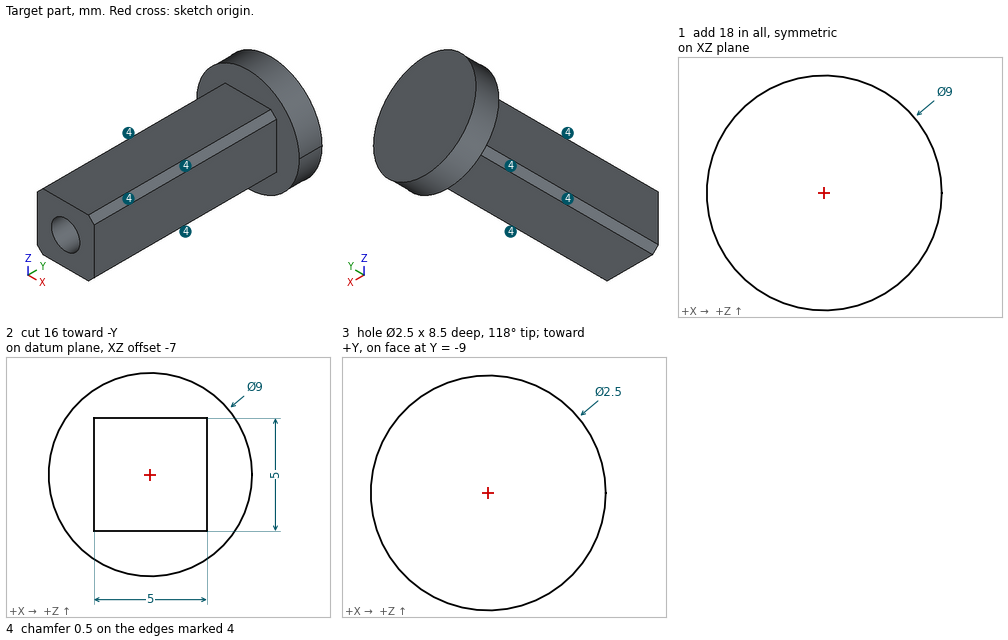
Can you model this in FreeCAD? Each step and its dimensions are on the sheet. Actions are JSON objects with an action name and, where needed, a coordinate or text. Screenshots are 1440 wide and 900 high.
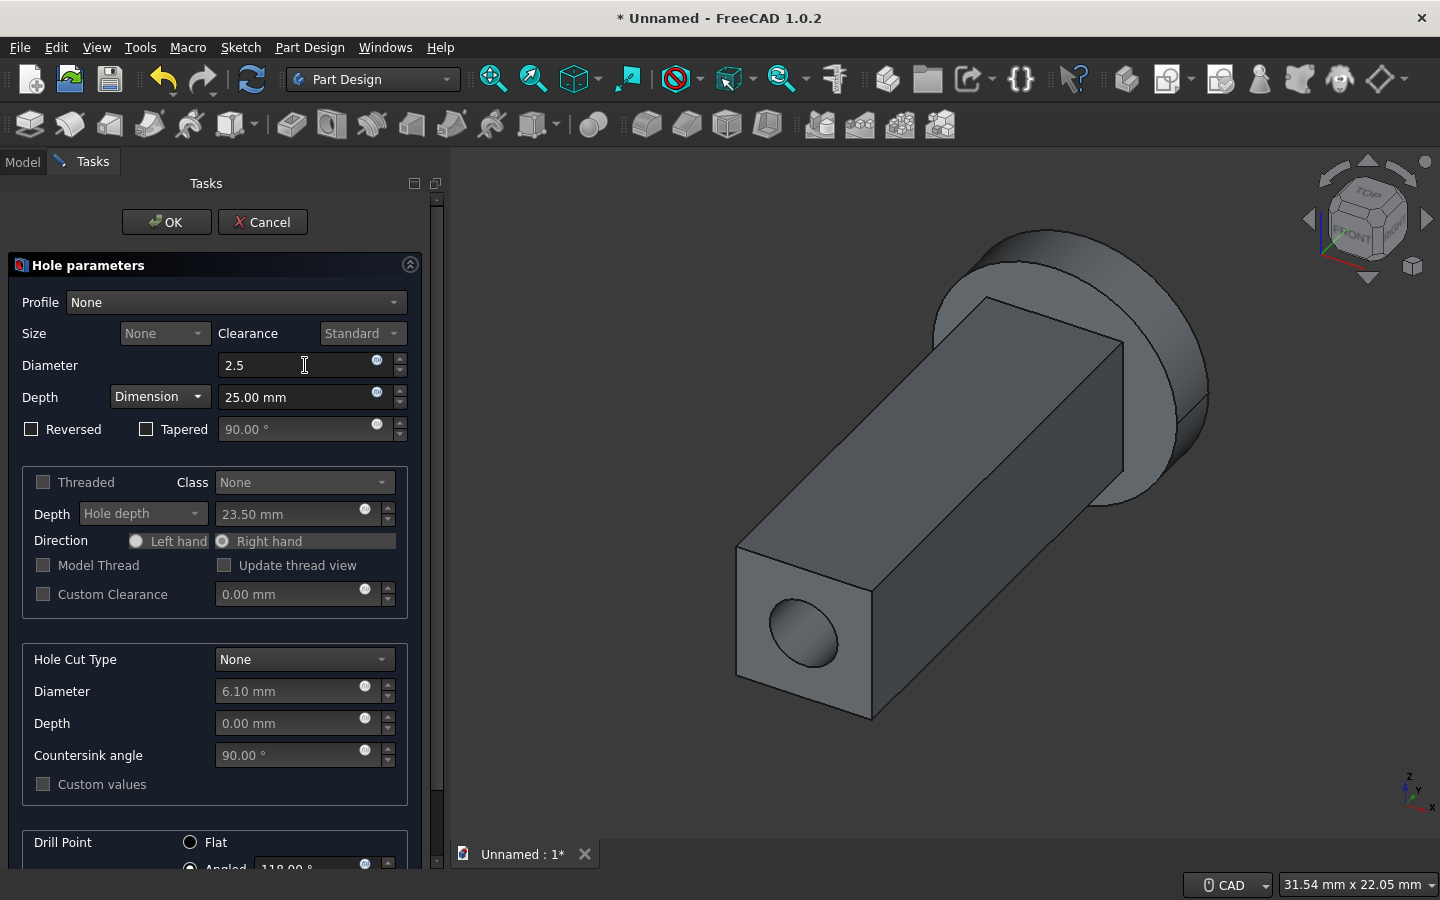
{"action": "triple_click", "coordinate": [305, 397]}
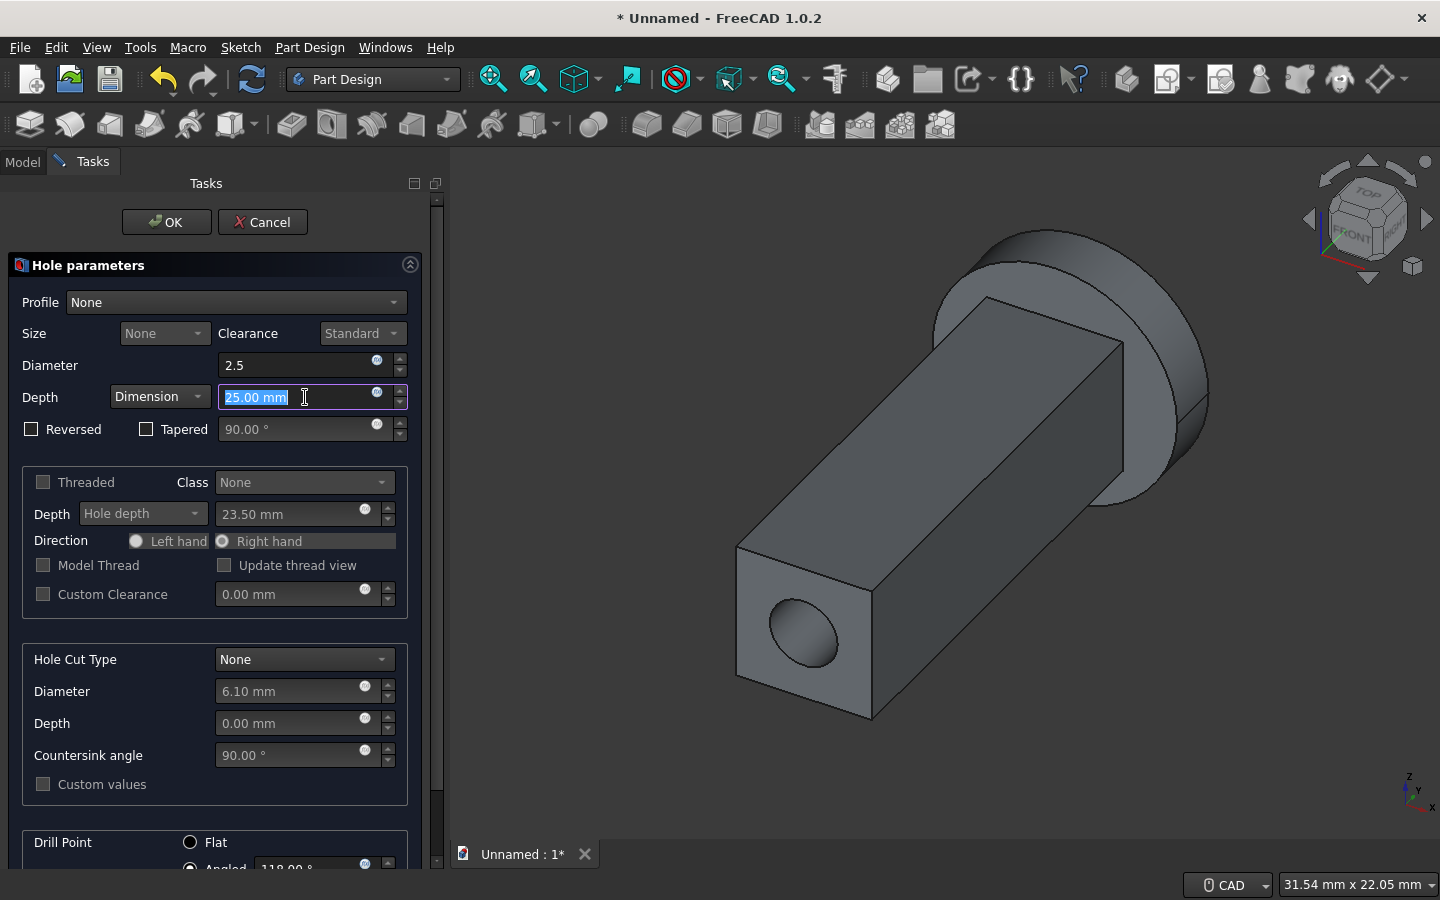
{"action": "type", "text": "8.5"}
{"action": "key", "text": "Tab"}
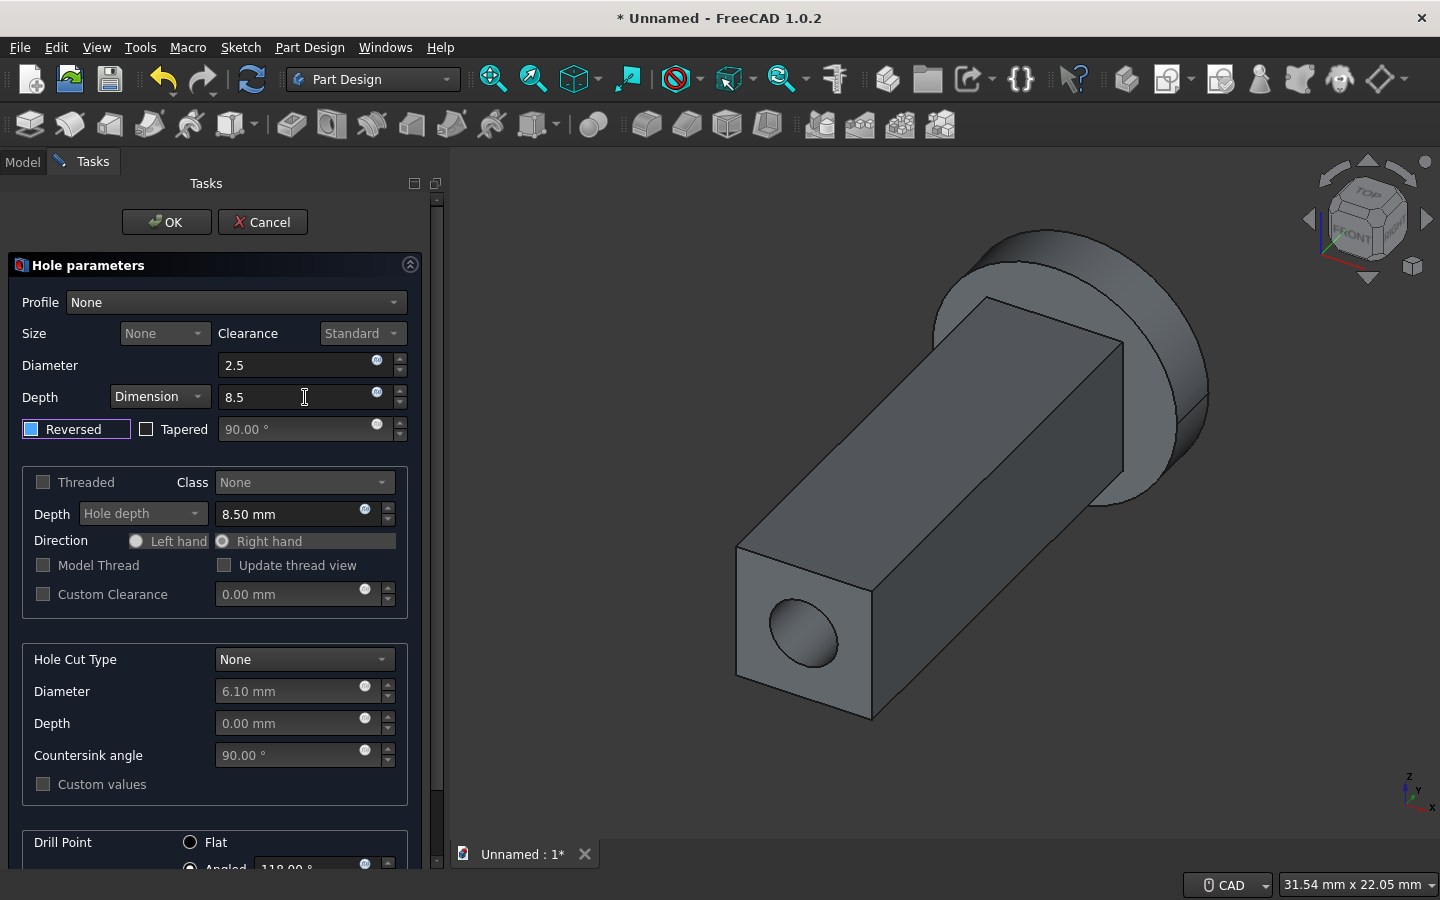
{"action": "left_click", "coordinate": [167, 222]}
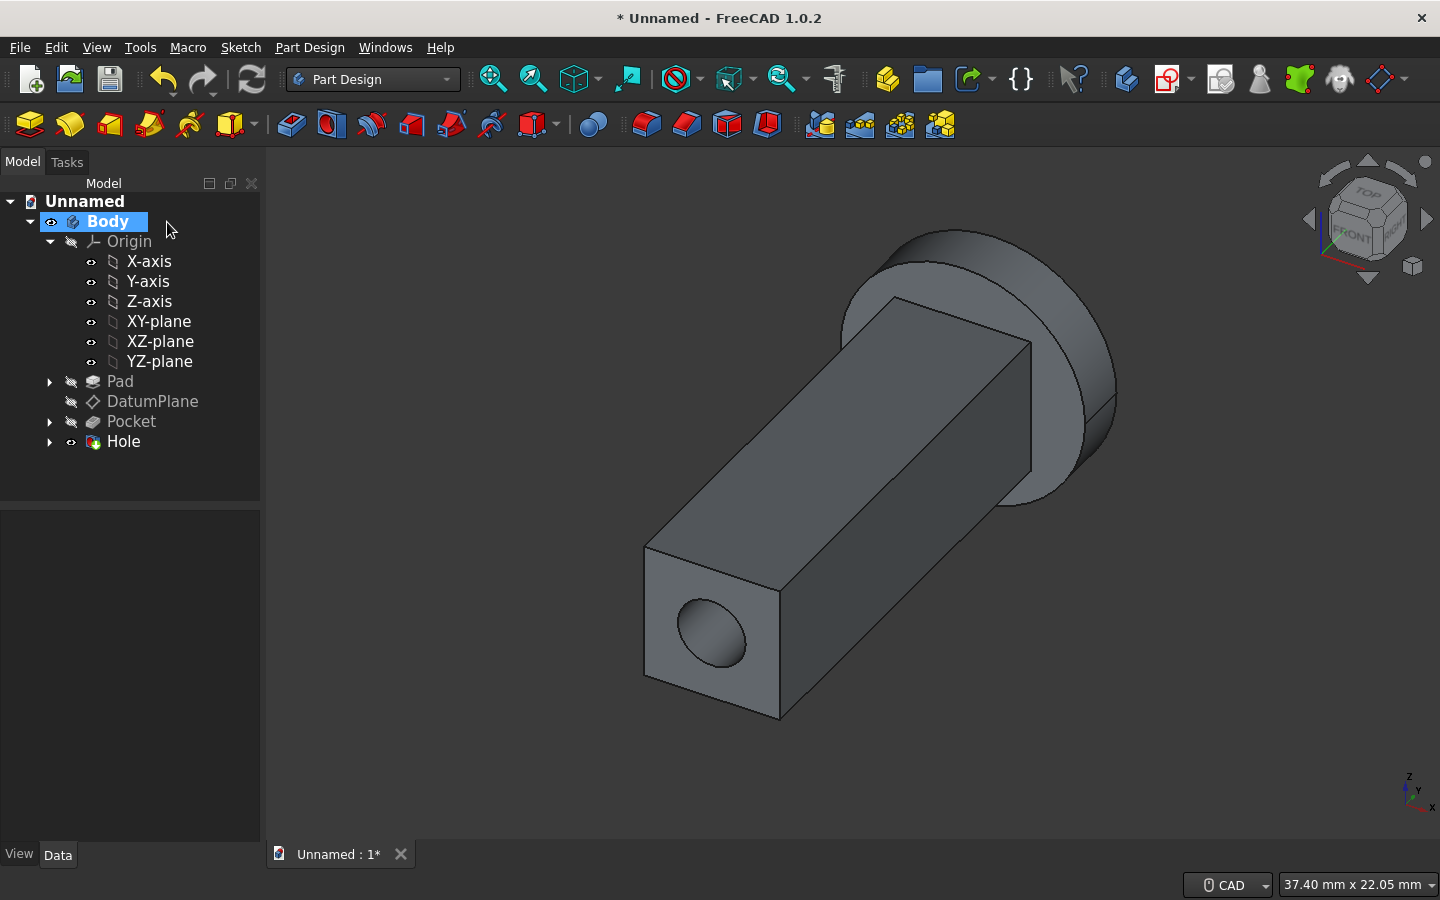
{"action": "left_click", "coordinate": [905, 466]}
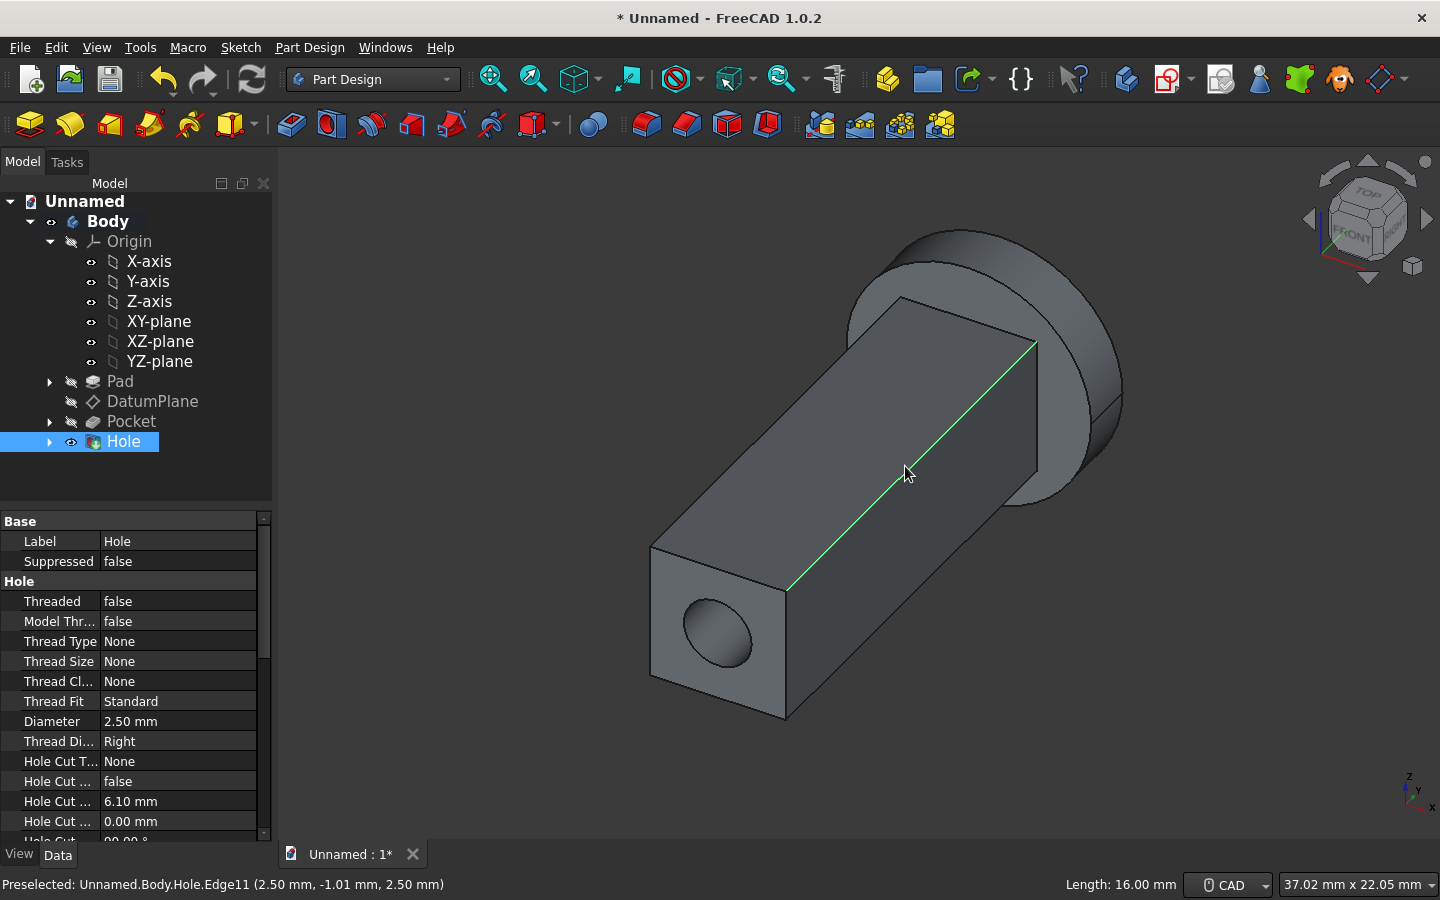
{"action": "key", "text": "0"}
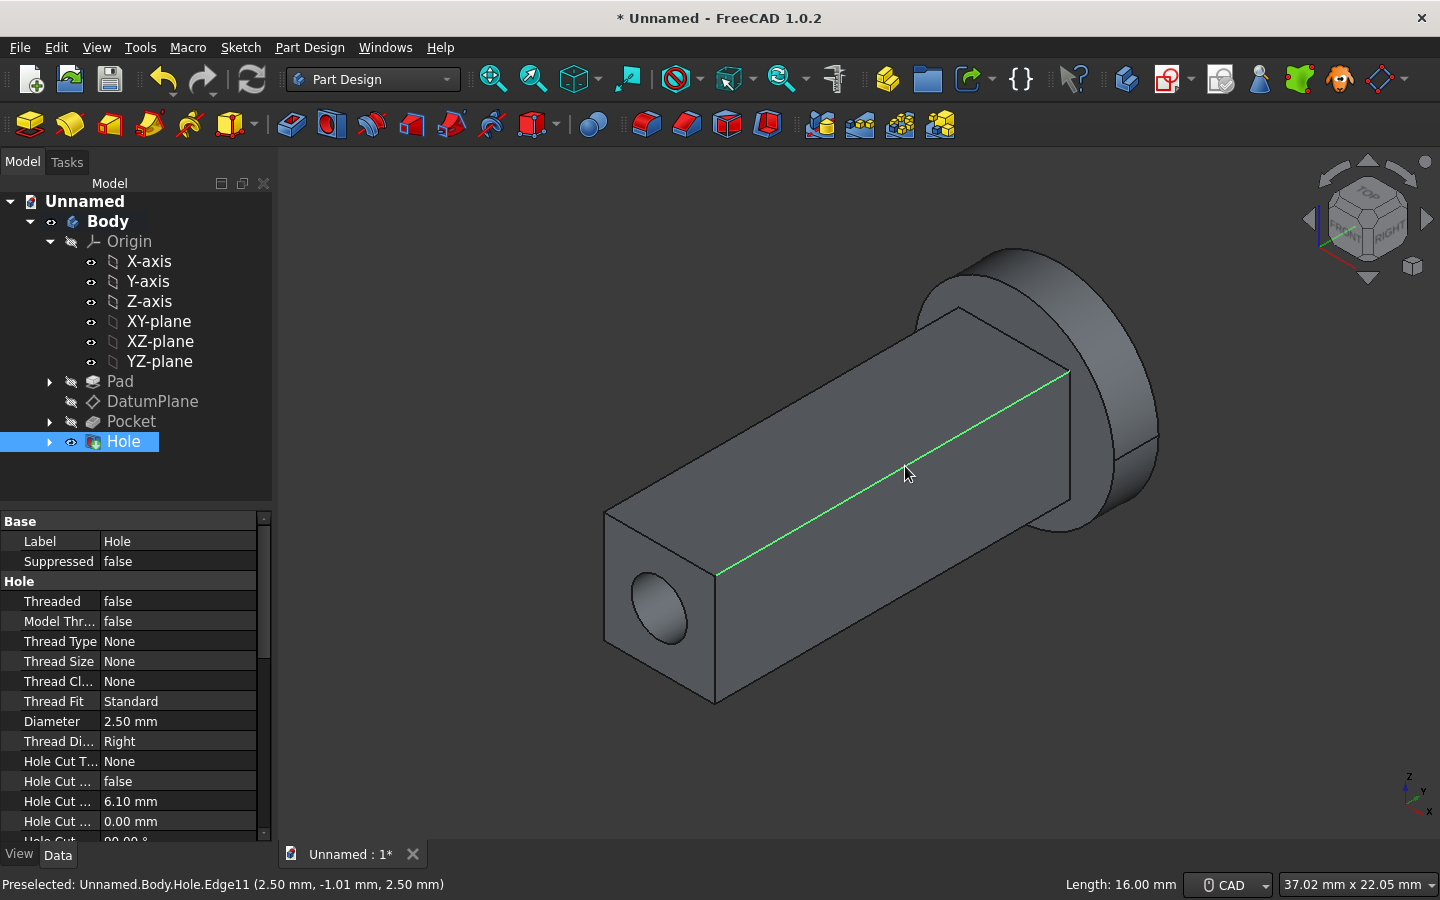
{"action": "key", "text": "2"}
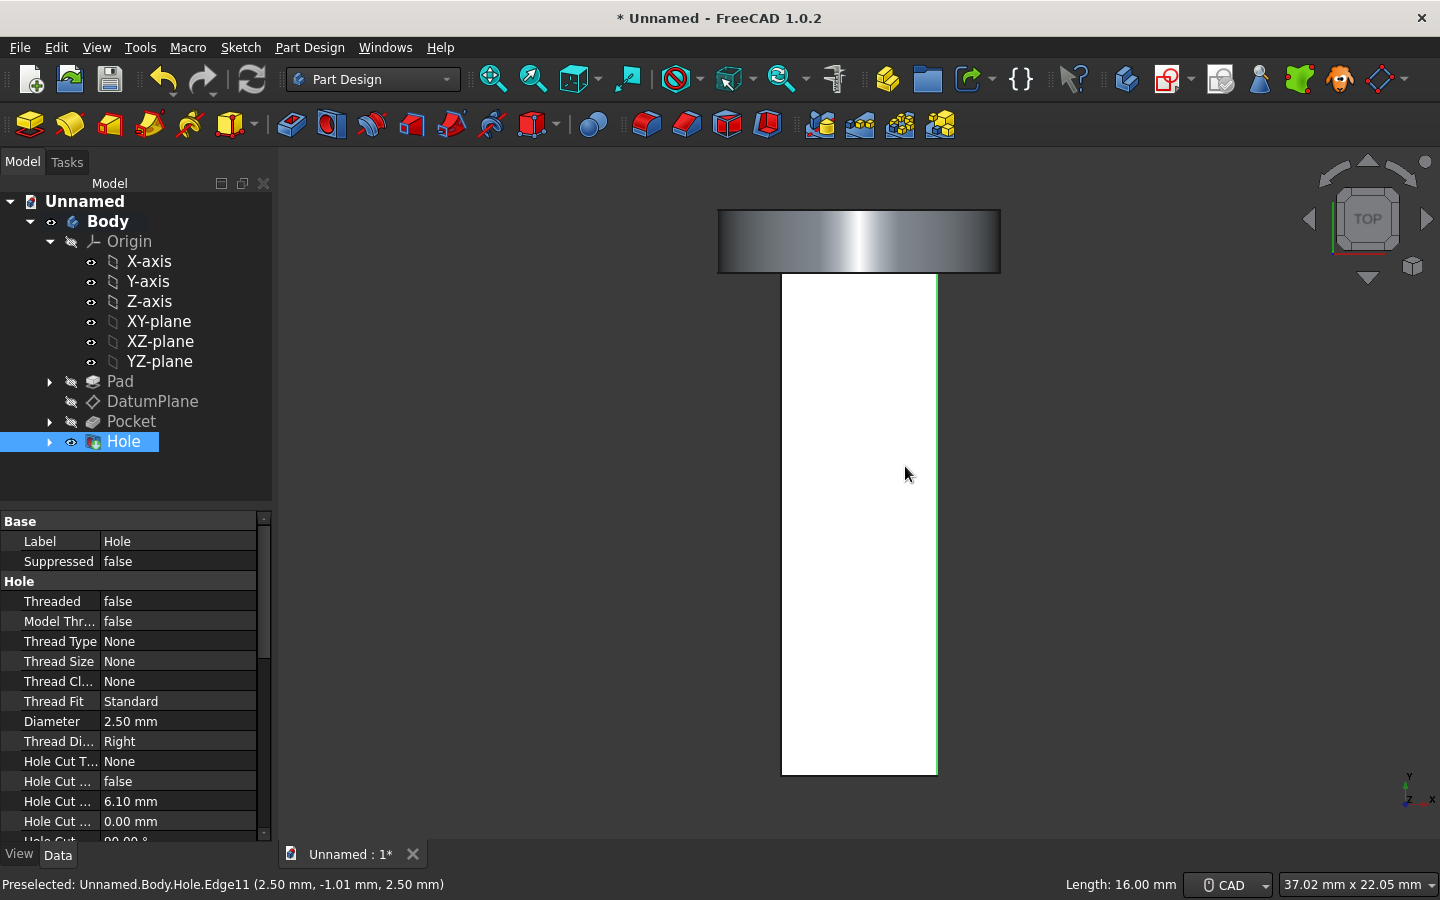
{"action": "left_click", "coordinate": [781, 523], "text": "ctrl"}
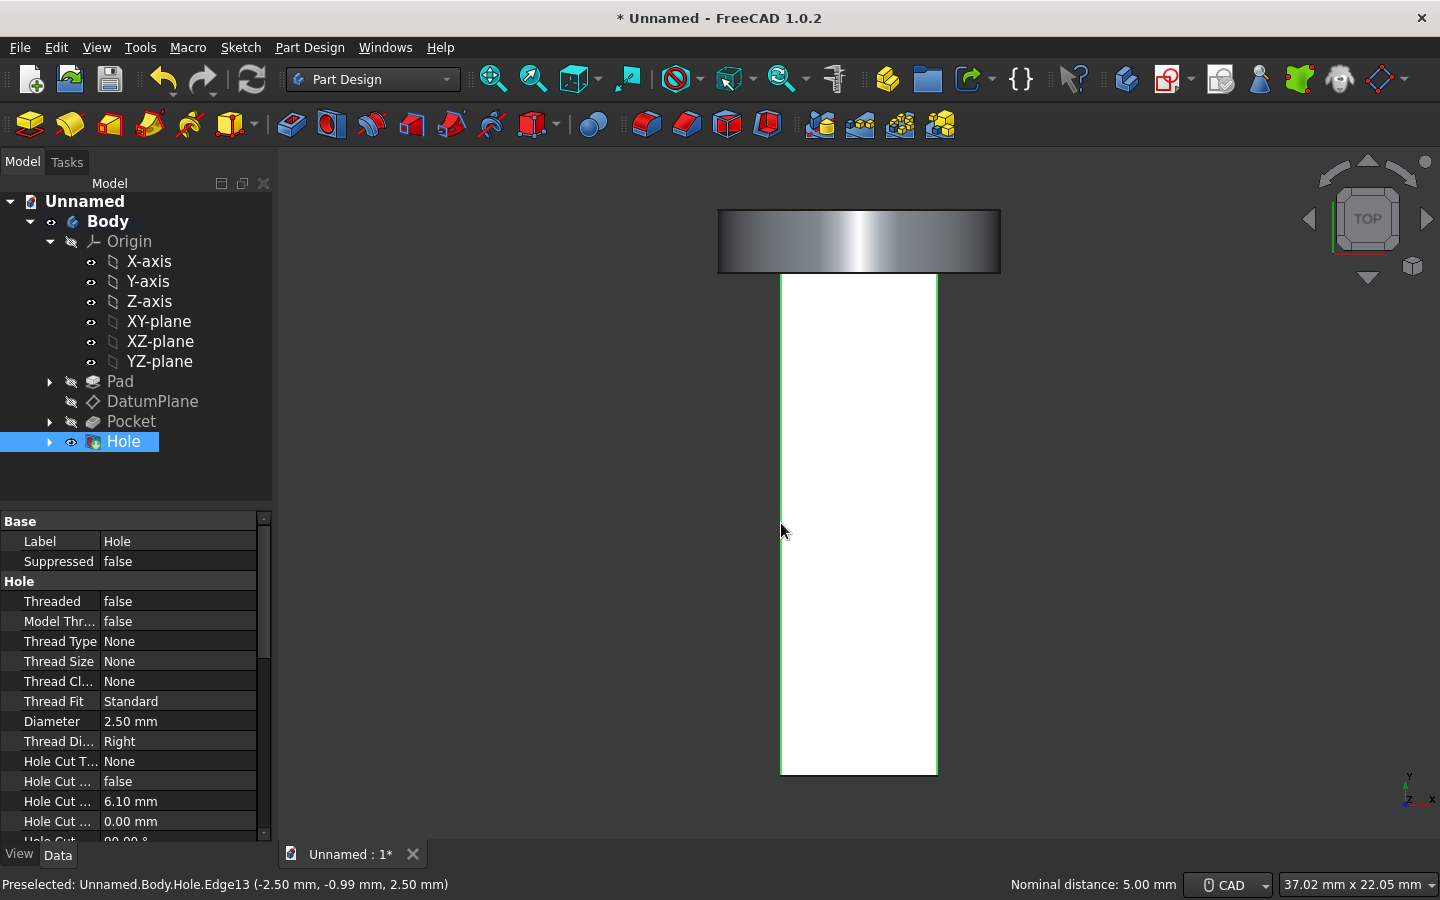
{"action": "key", "text": "1"}